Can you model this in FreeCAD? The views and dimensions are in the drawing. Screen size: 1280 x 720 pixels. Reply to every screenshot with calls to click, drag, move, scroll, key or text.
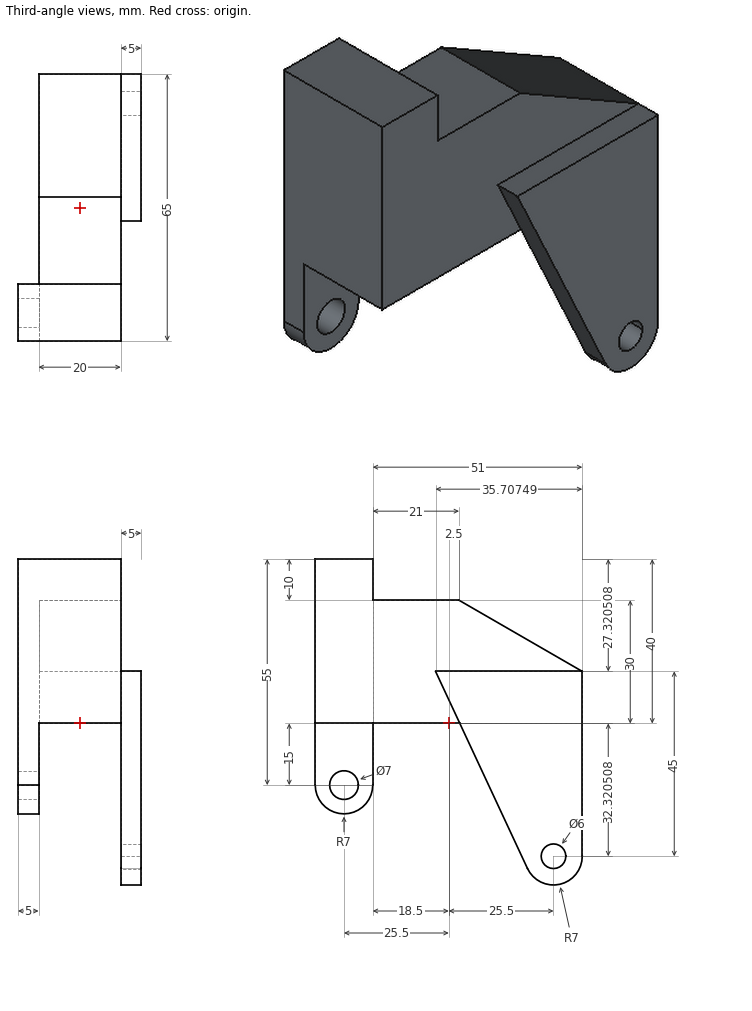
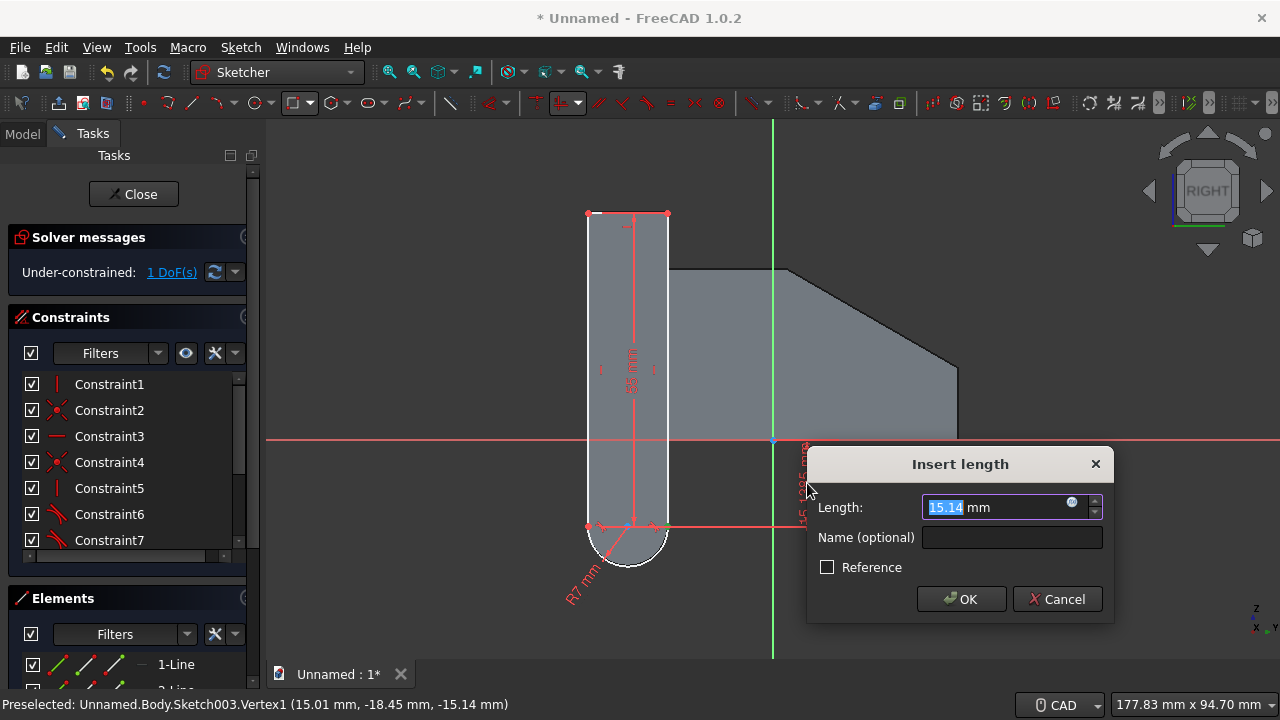
text(15)
key(Return)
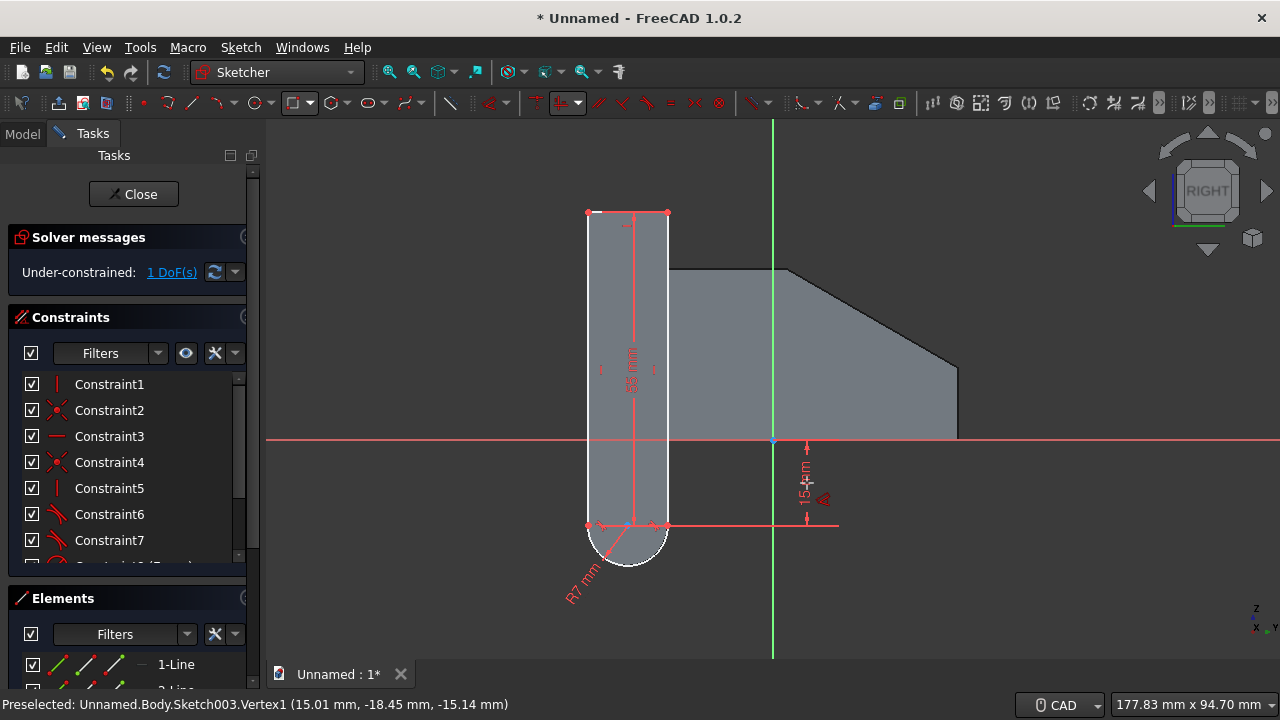
click(668, 526)
click(720, 560)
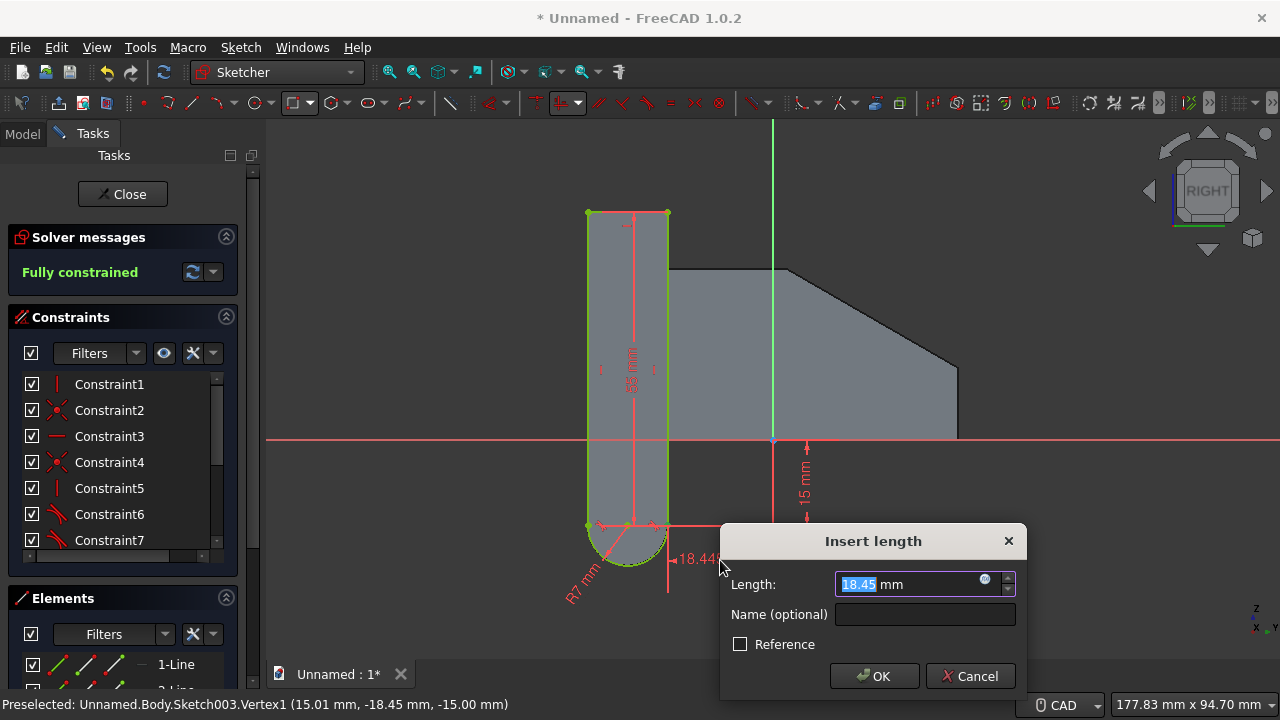
text(18.5)
key(Return)
key(Escape)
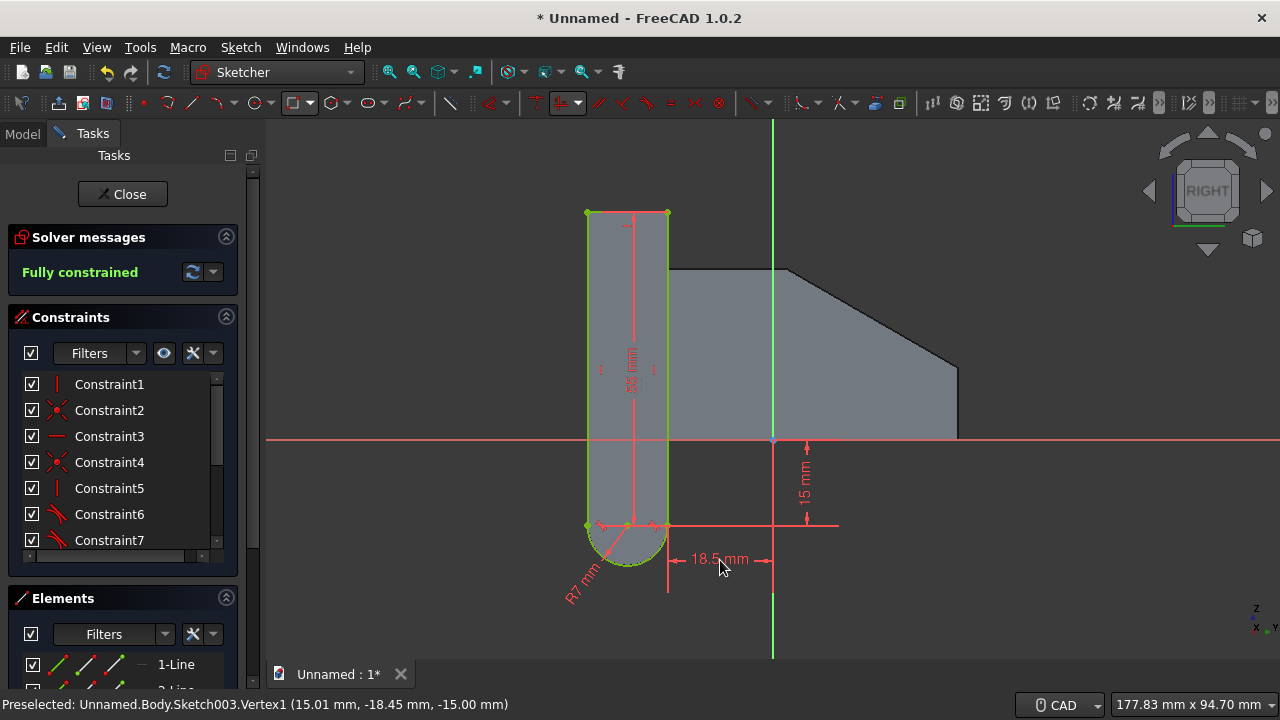
click(123, 194)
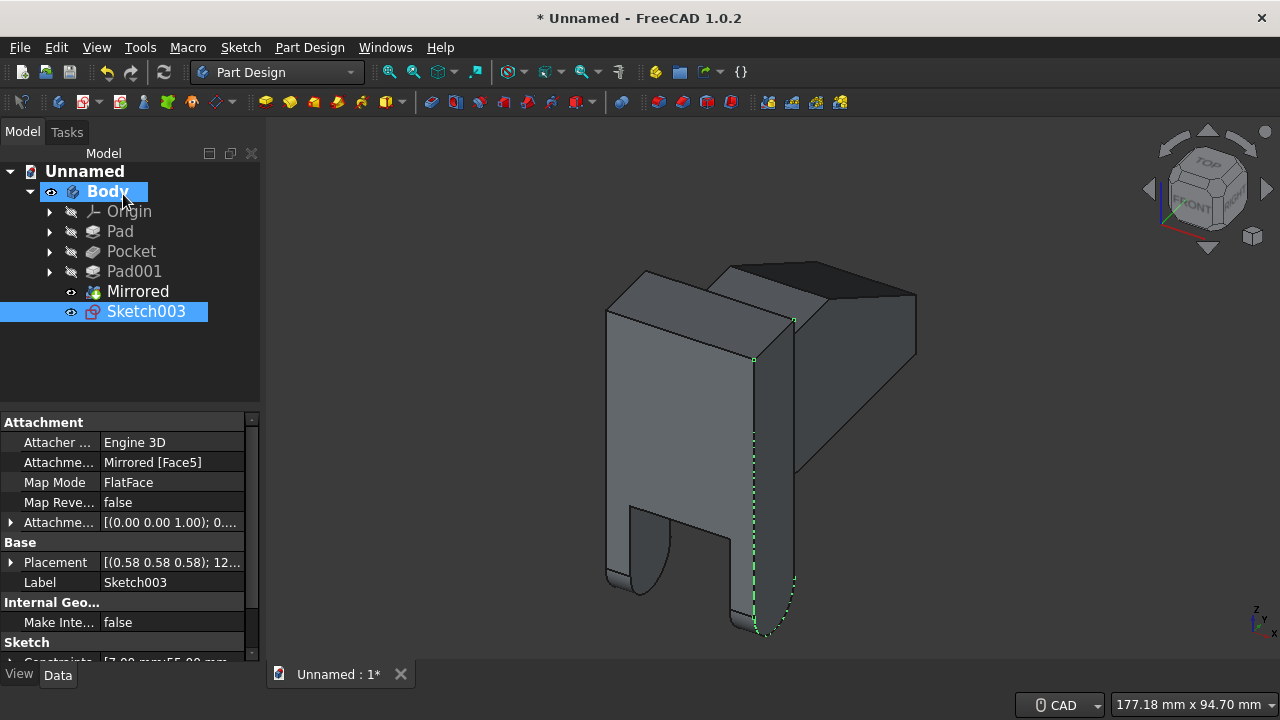
click(432, 102)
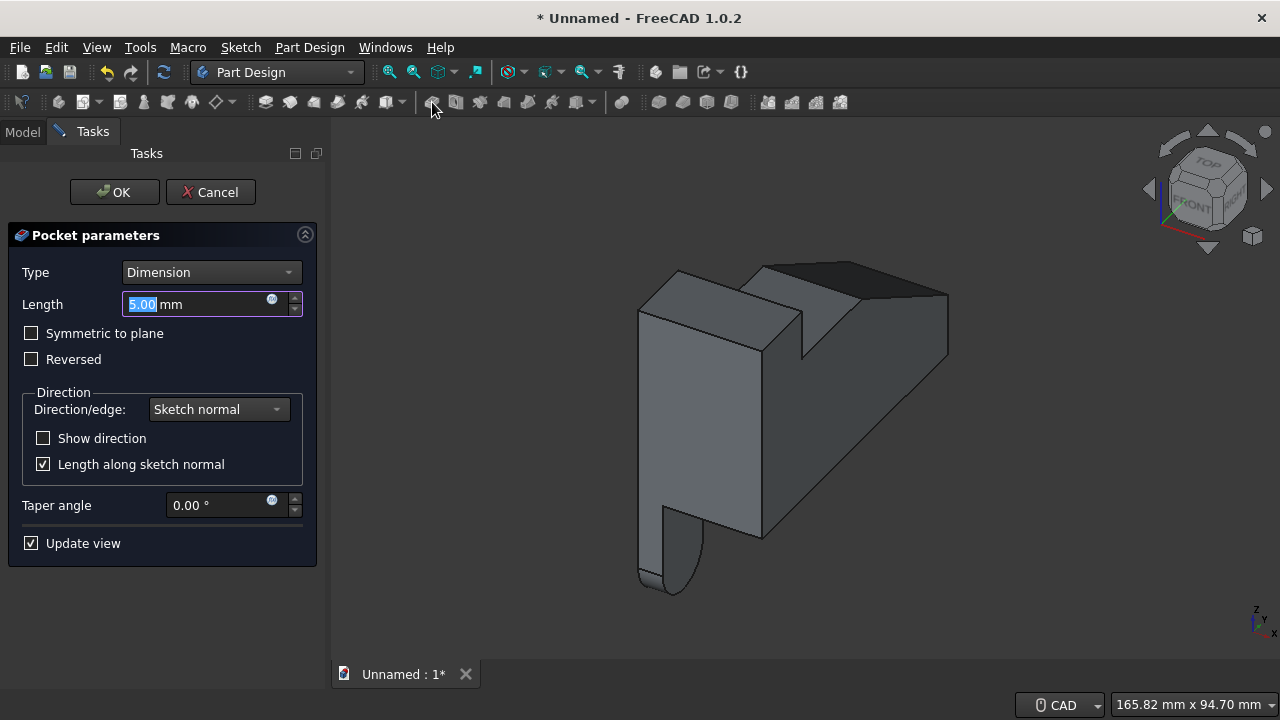
click(212, 272)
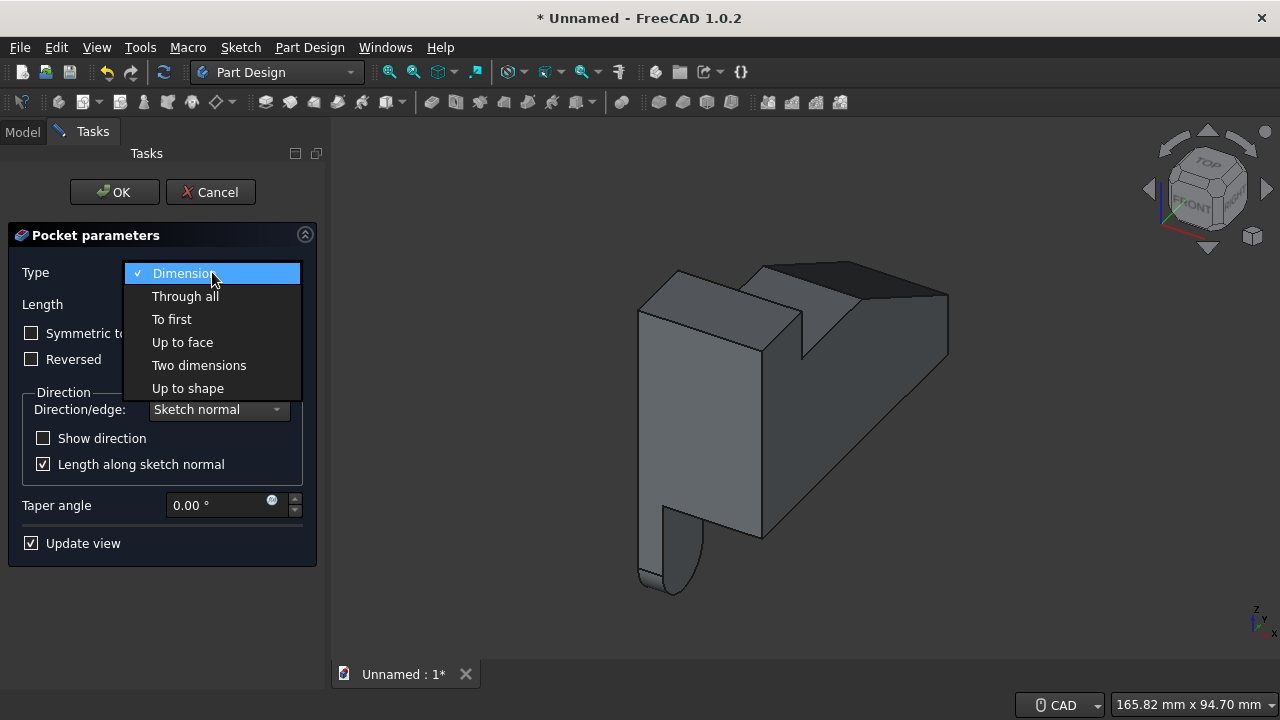
click(212, 366)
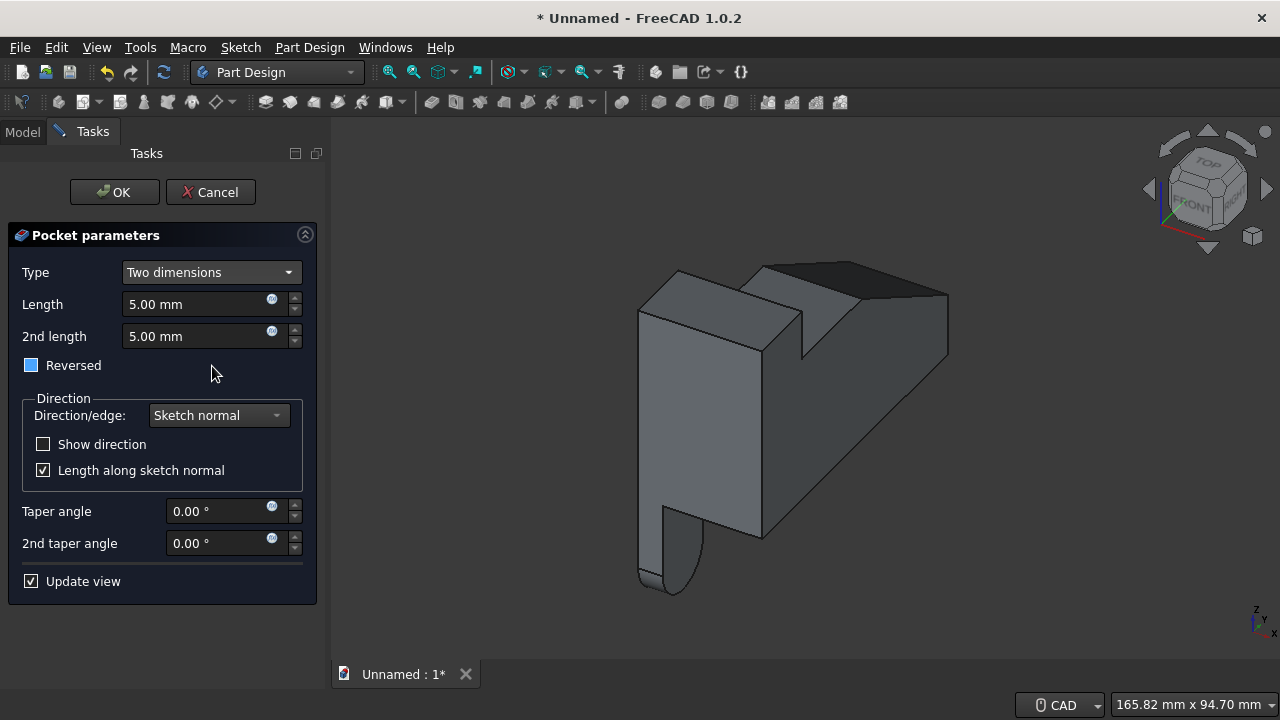
triple_click(204, 304)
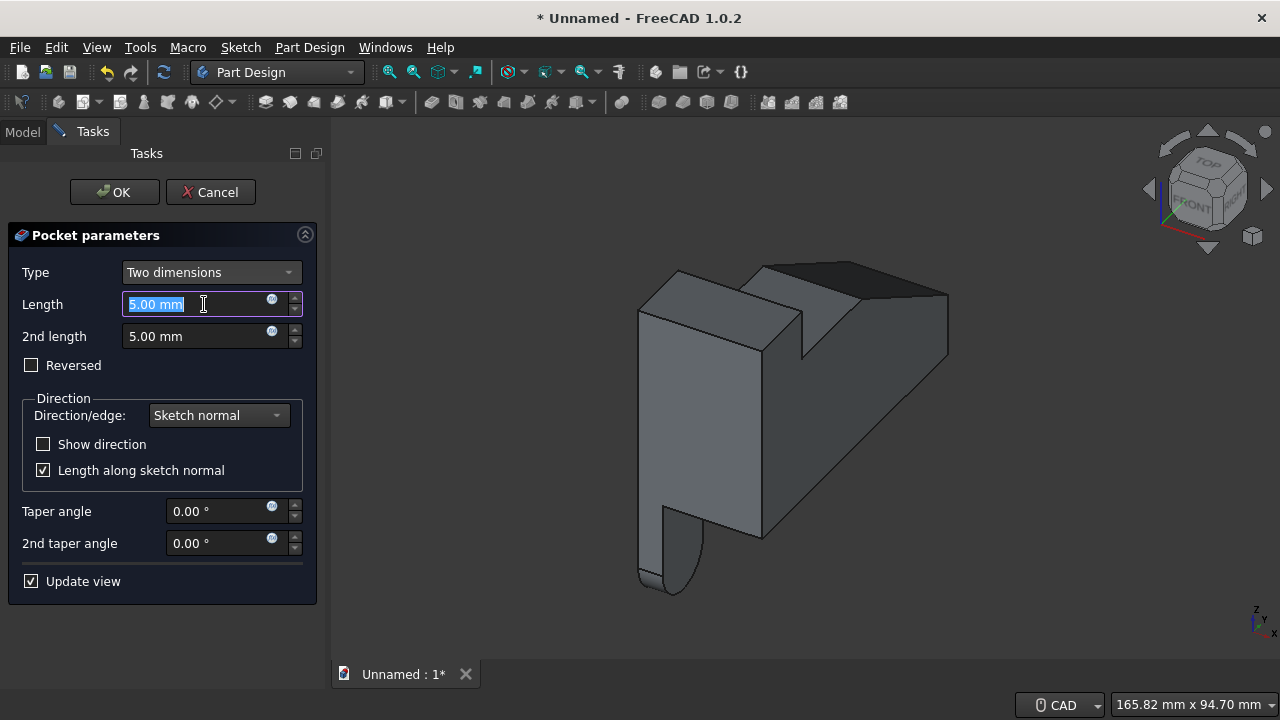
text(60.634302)
key(Tab)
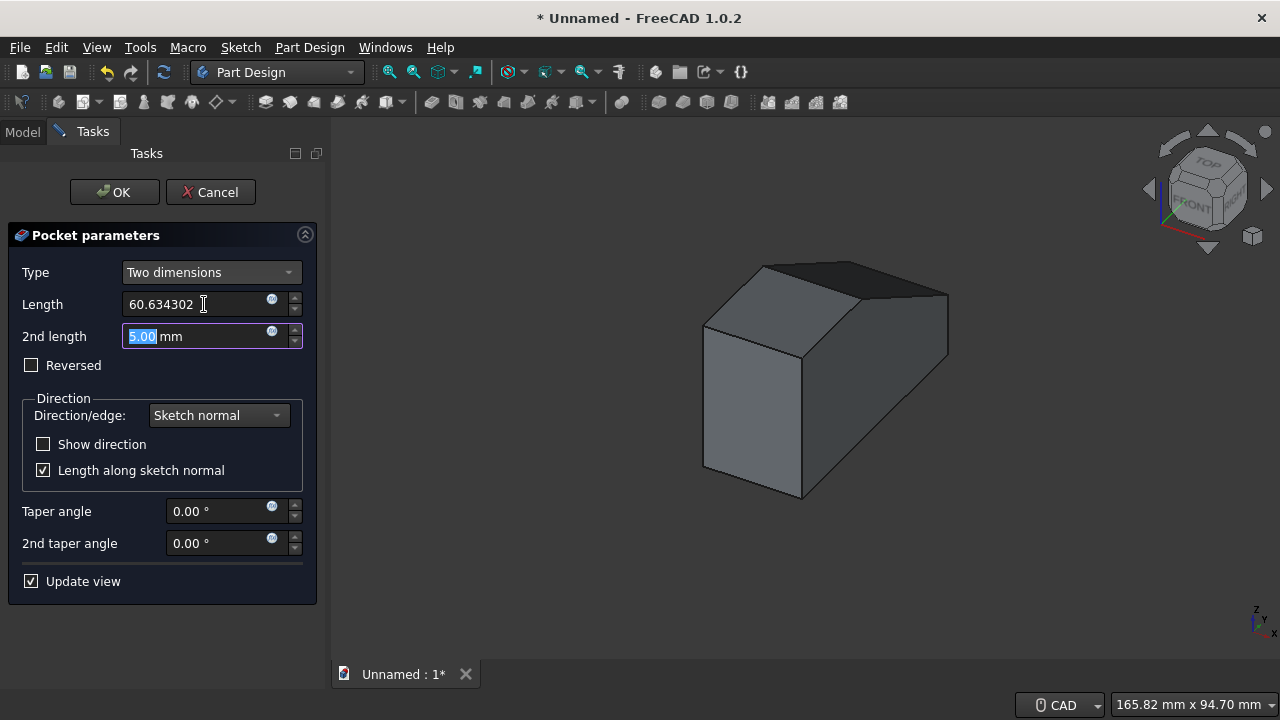
text(5)
key(Tab)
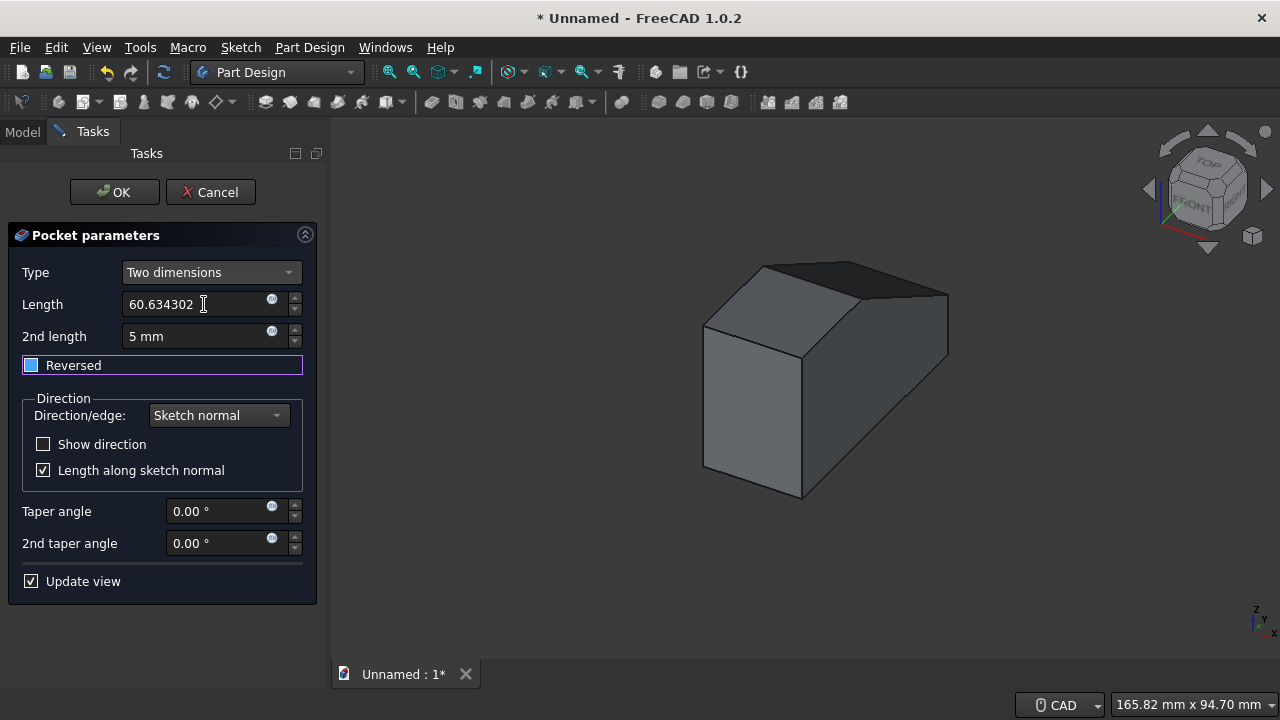
click(30, 365)